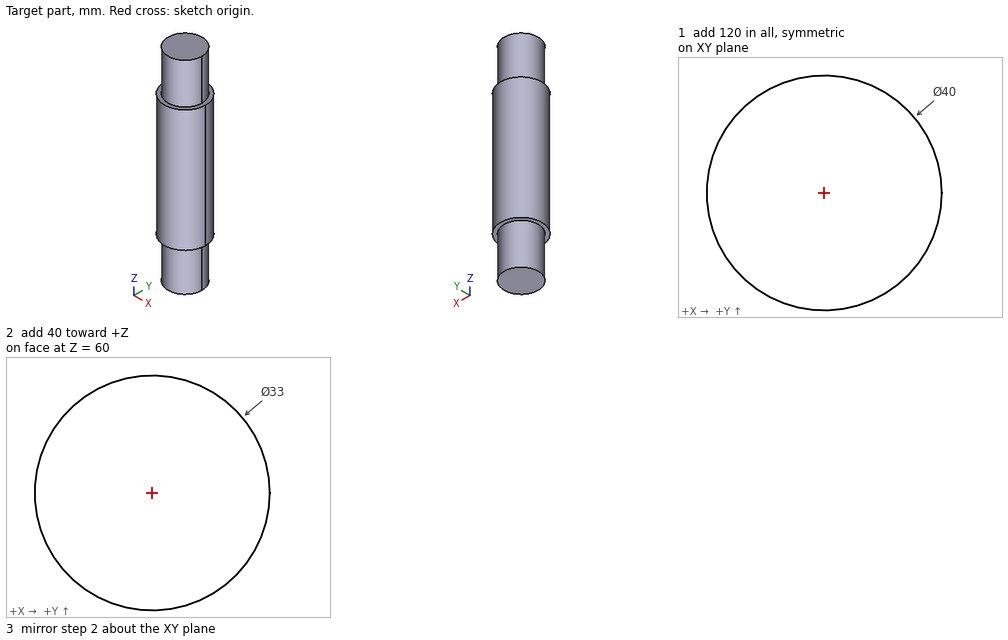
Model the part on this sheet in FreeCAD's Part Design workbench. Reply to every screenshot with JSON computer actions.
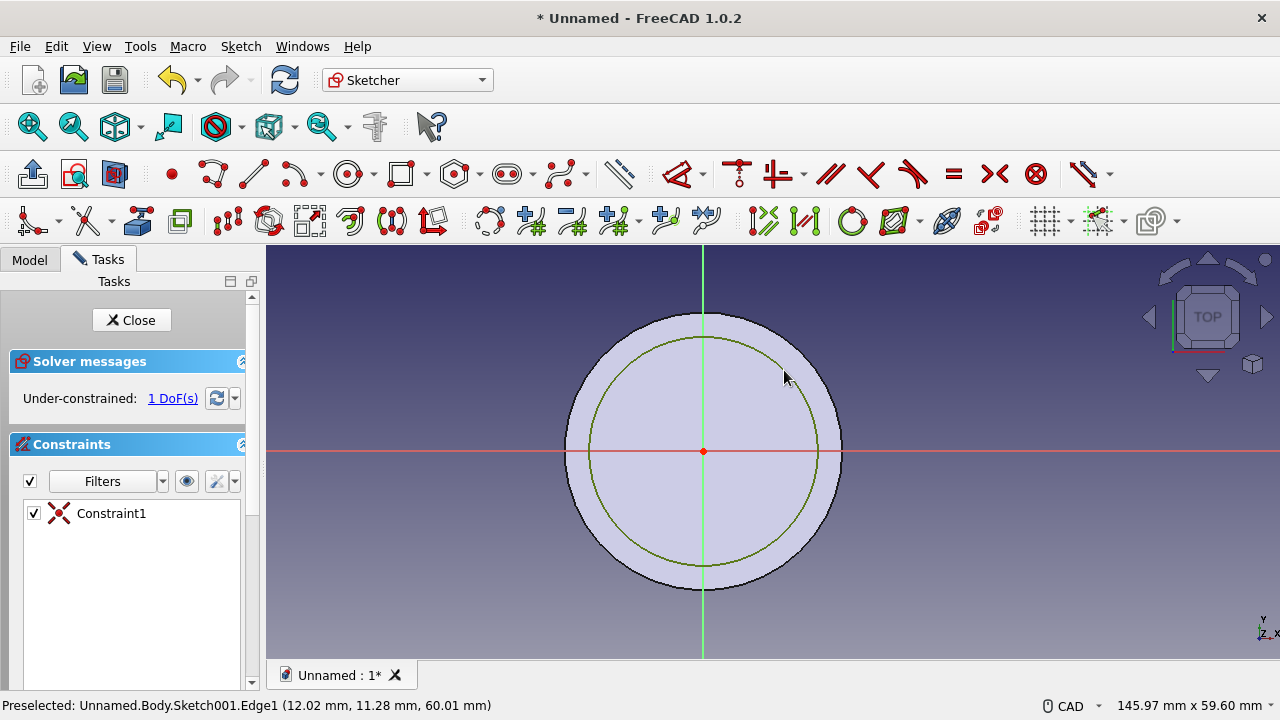
{"action": "key", "text": "k o"}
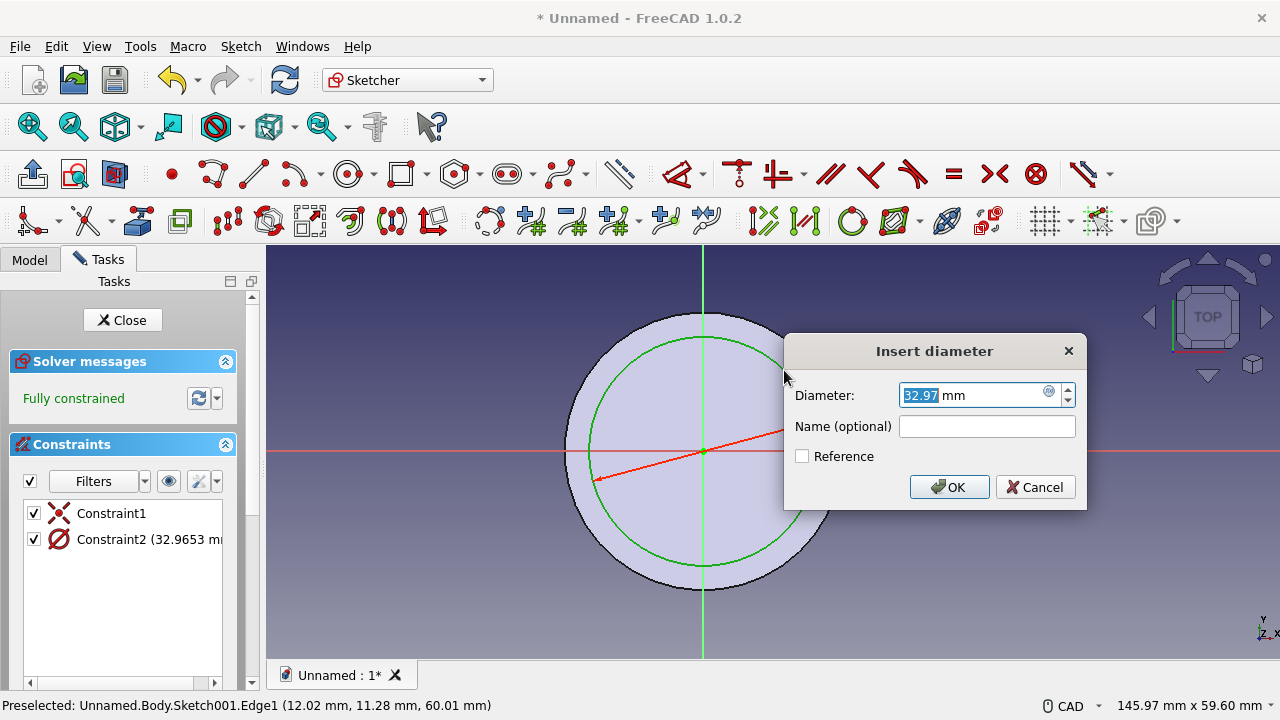
{"action": "type", "text": "33"}
{"action": "key", "text": "Return"}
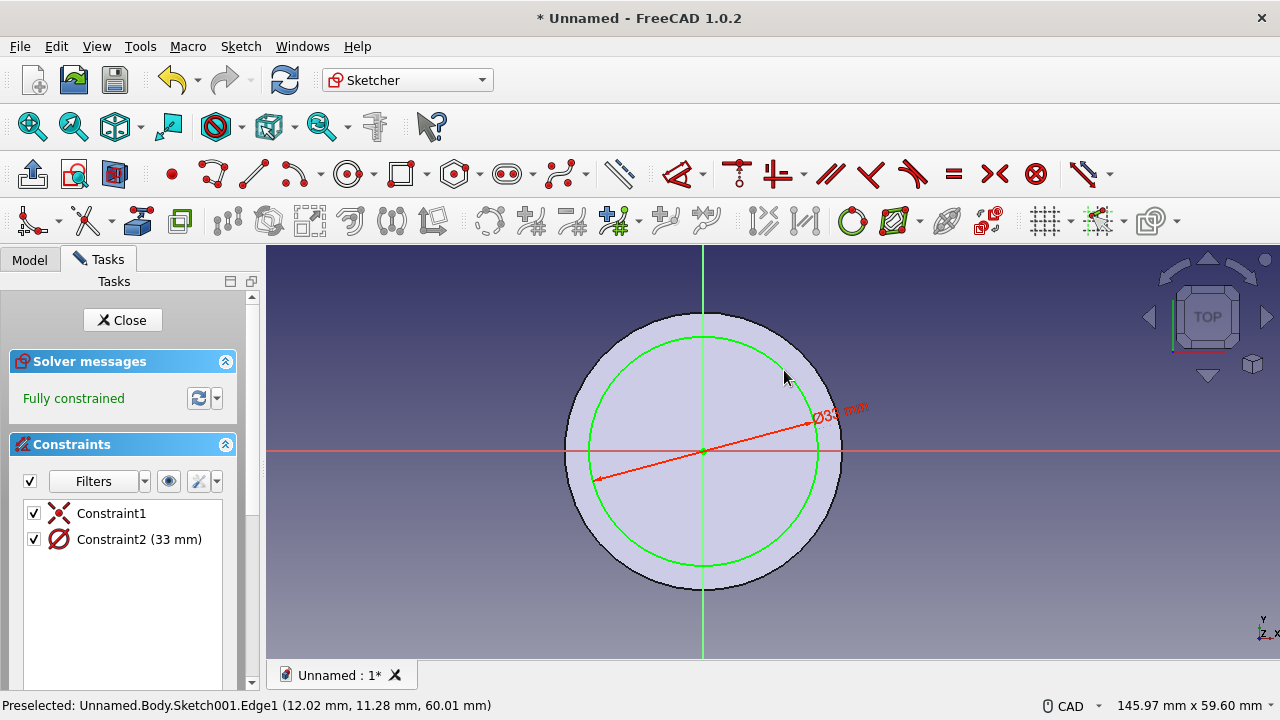
{"action": "left_click", "coordinate": [123, 320]}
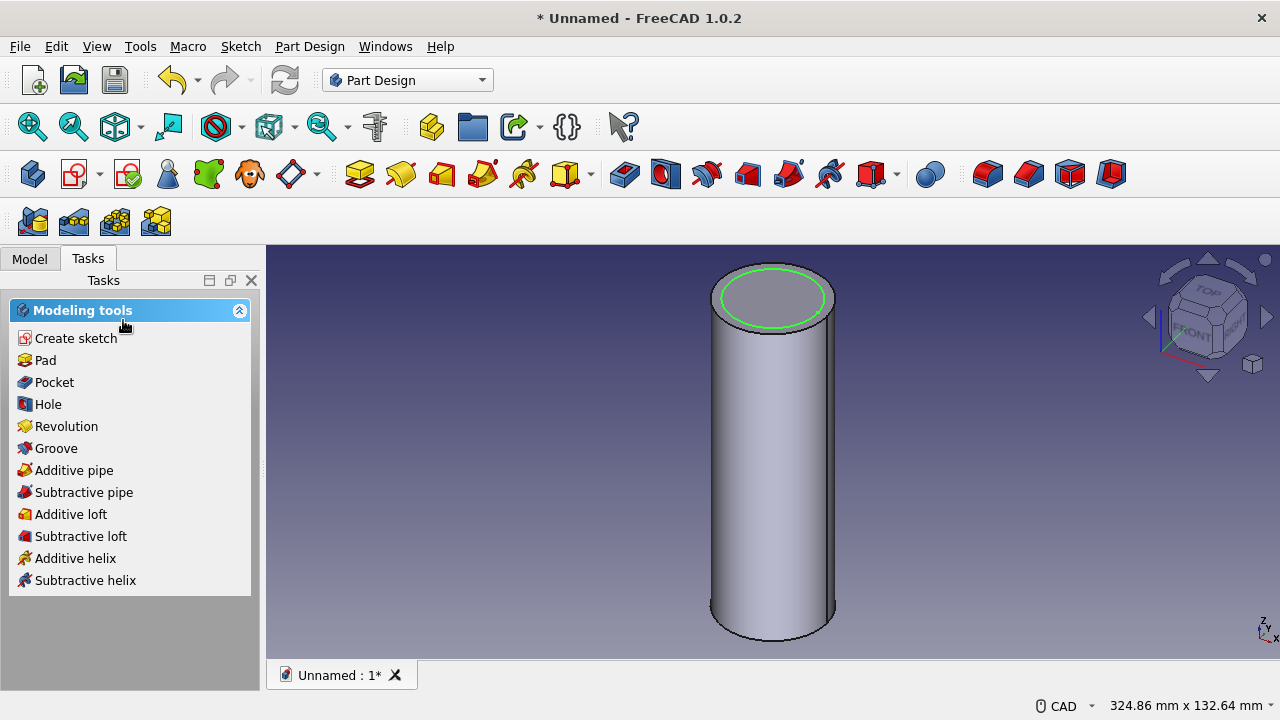
{"action": "left_click", "coordinate": [360, 174]}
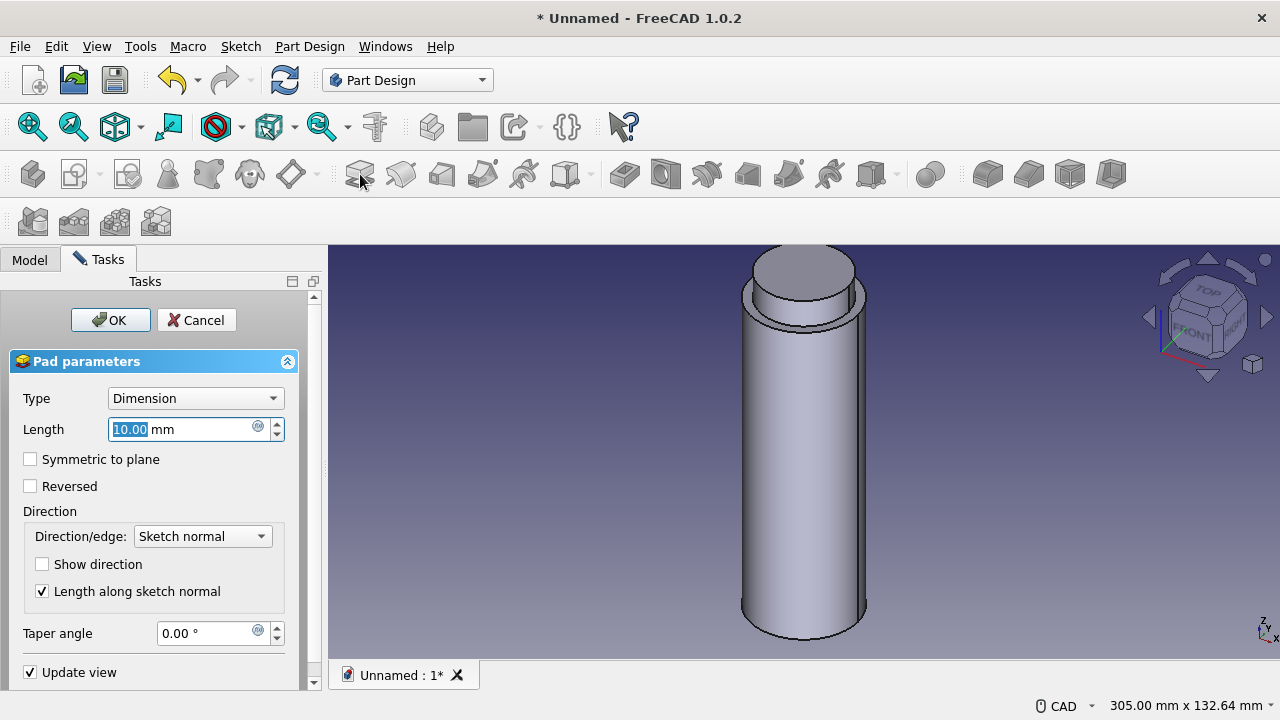
{"action": "type", "text": "40"}
{"action": "key", "text": "Tab"}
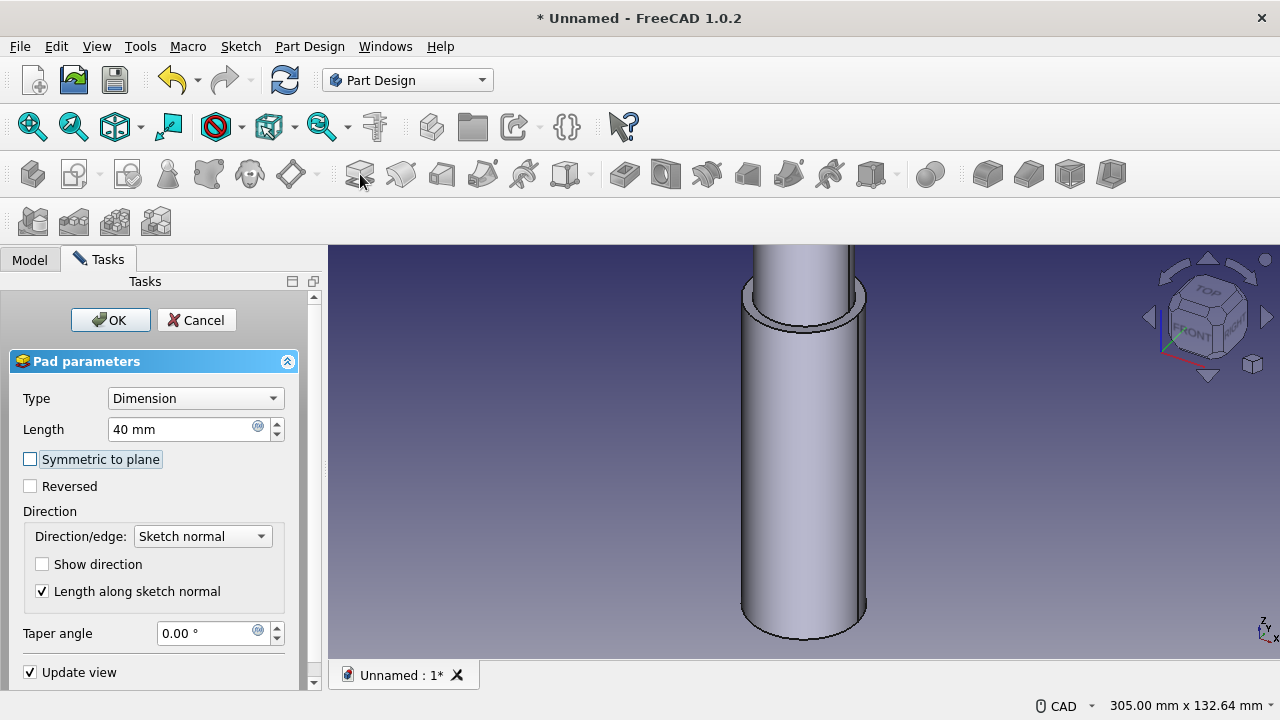
{"action": "left_click", "coordinate": [111, 320]}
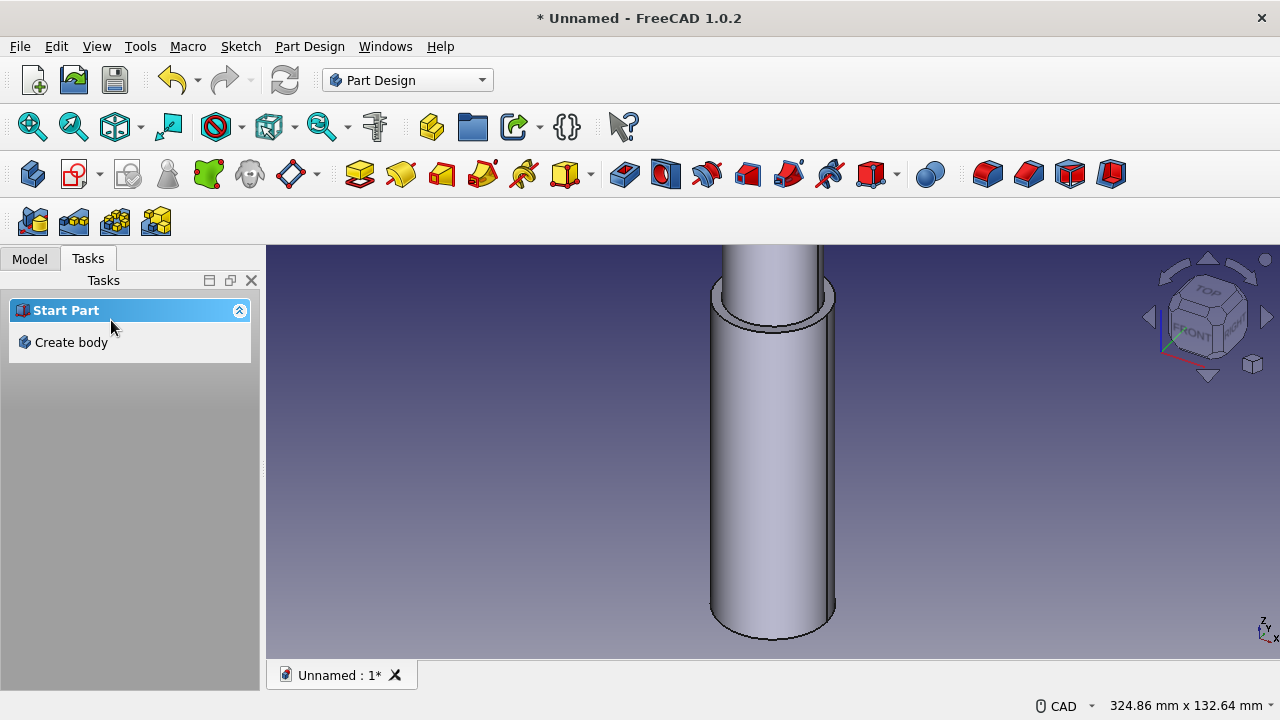
{"action": "left_click", "coordinate": [33, 128]}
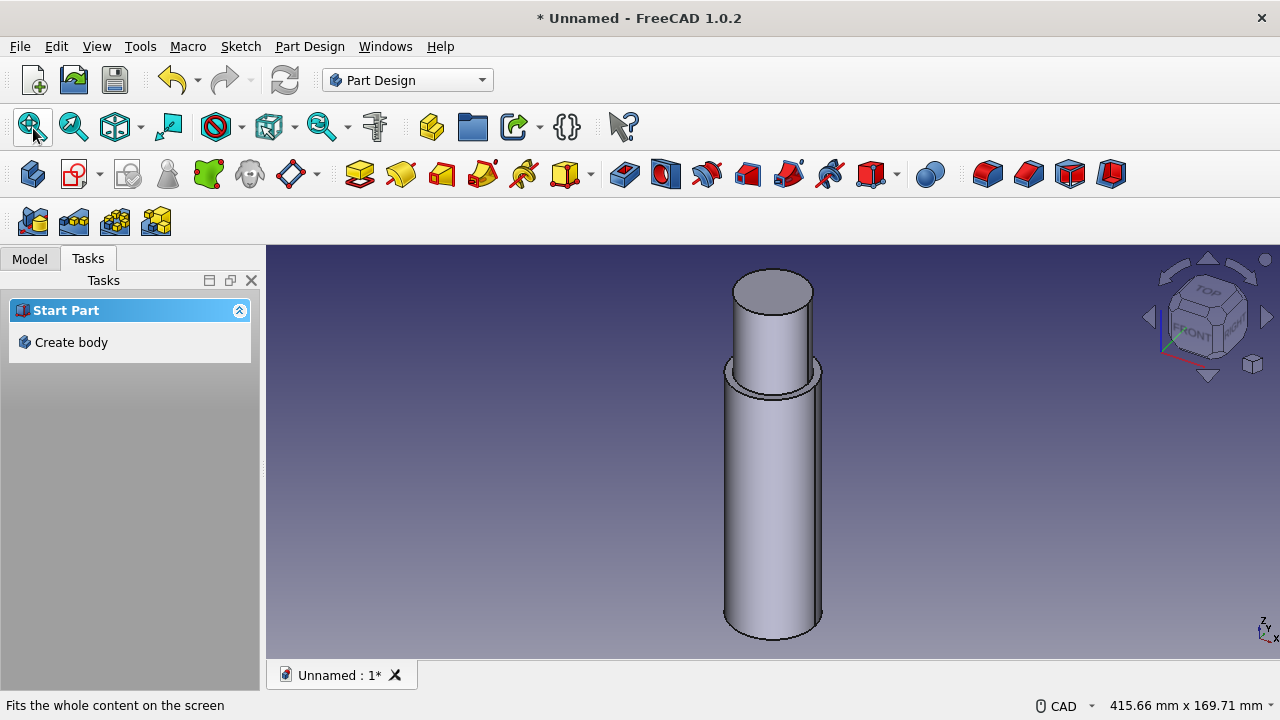
{"action": "left_click", "coordinate": [30, 258]}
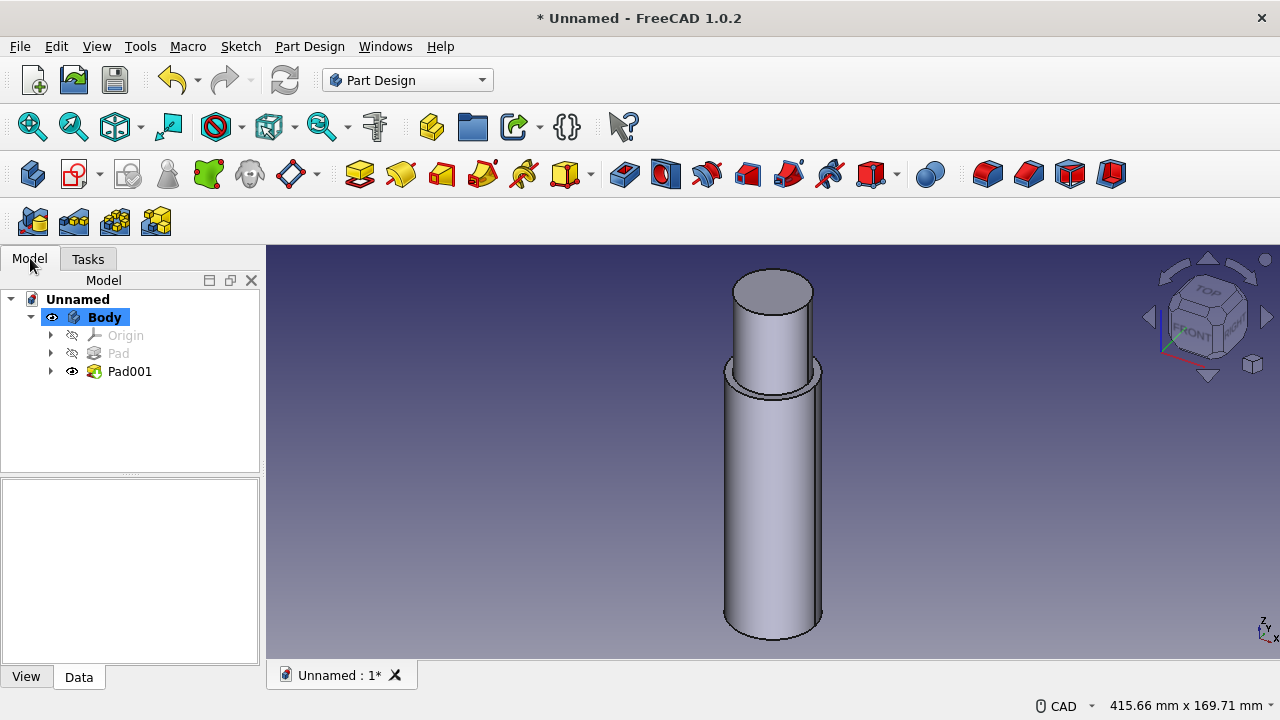
{"action": "left_click", "coordinate": [117, 371]}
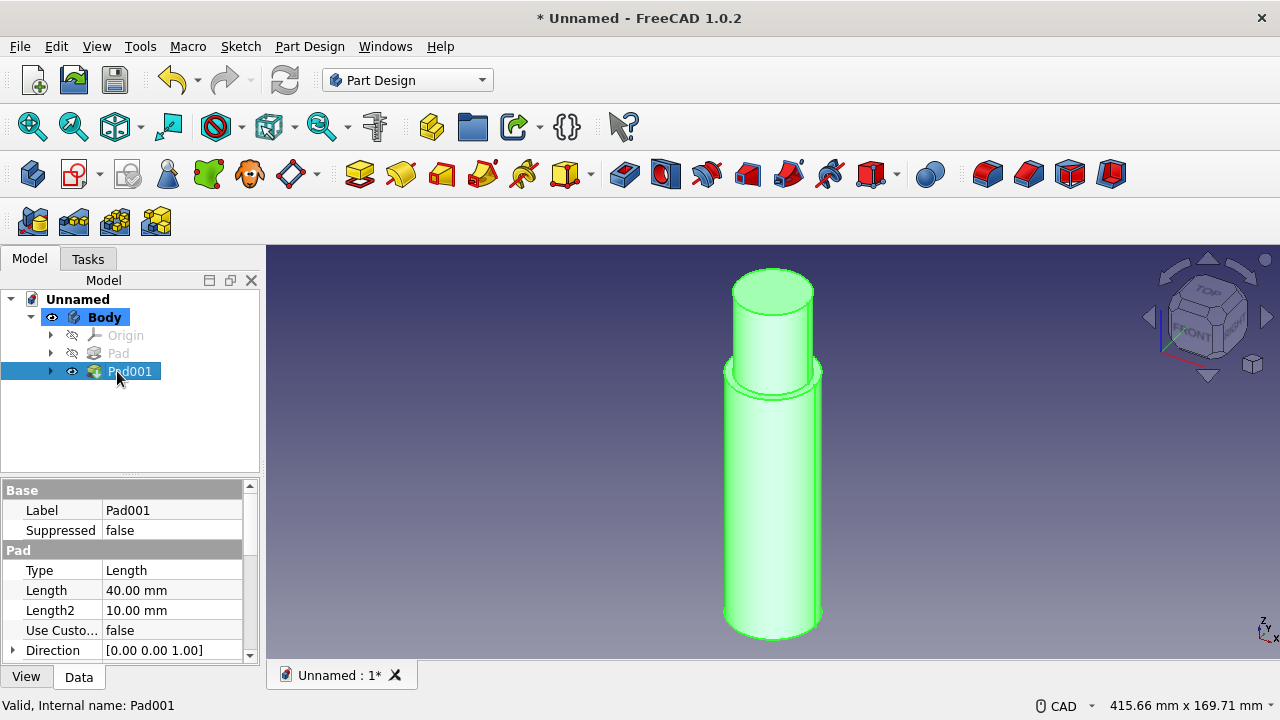
{"action": "left_click", "coordinate": [33, 222]}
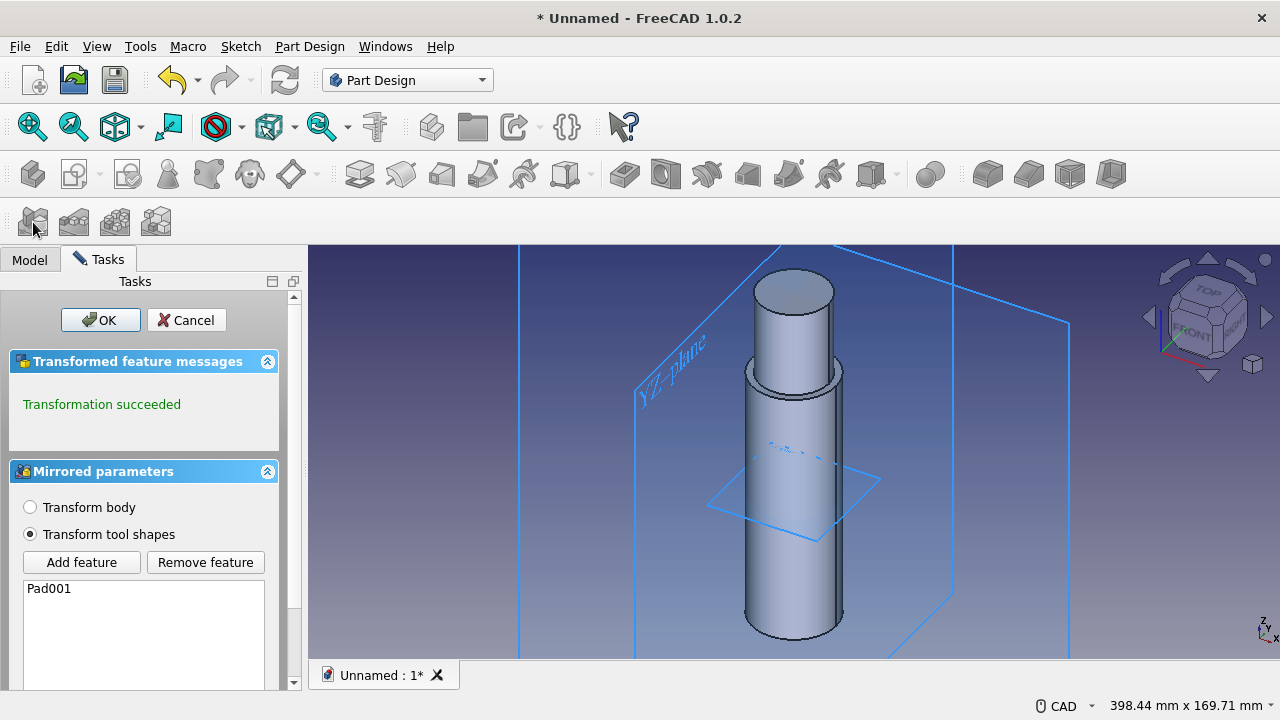
{"action": "scroll", "coordinate": [294, 490], "scroll_direction": "down", "scroll_amount": 2}